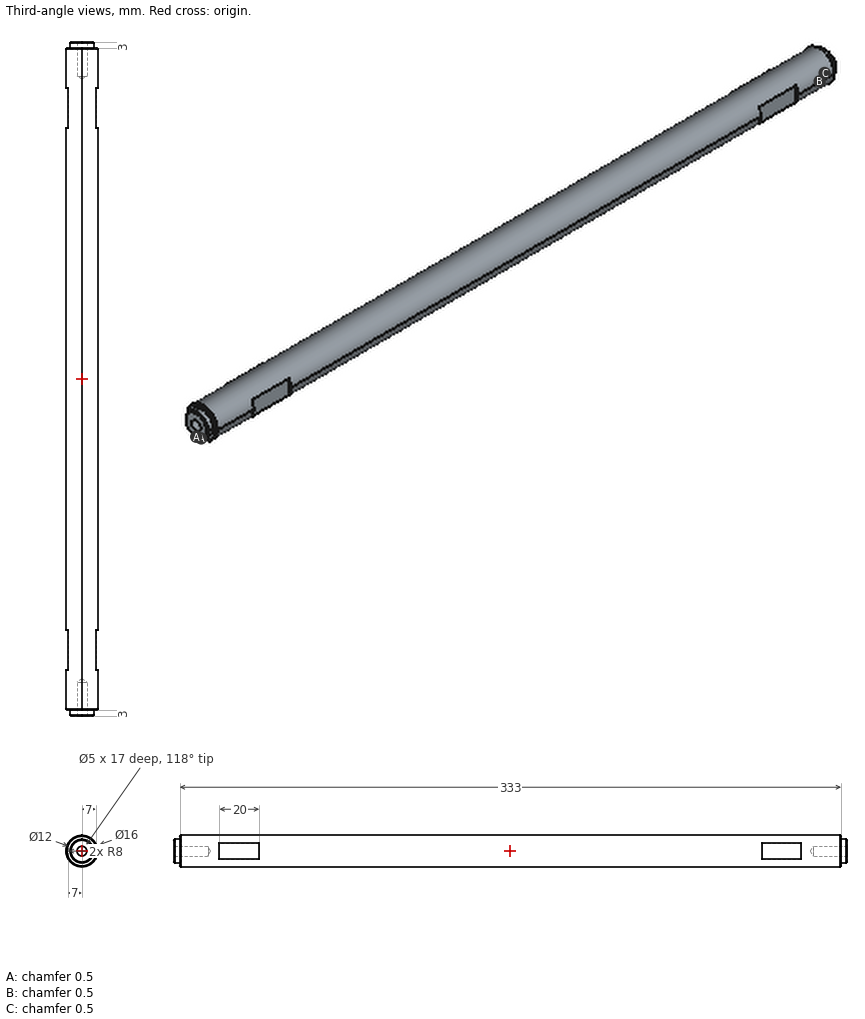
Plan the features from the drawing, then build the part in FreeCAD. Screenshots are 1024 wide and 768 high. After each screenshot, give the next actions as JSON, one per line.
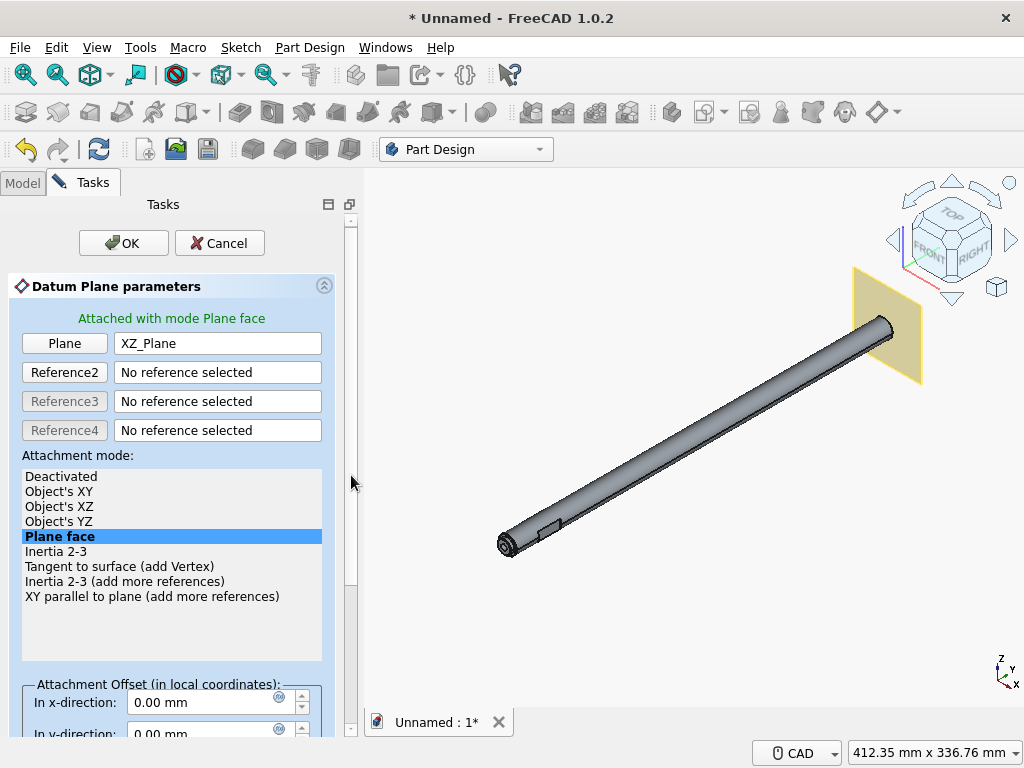
{"action": "left_click", "coordinate": [124, 243]}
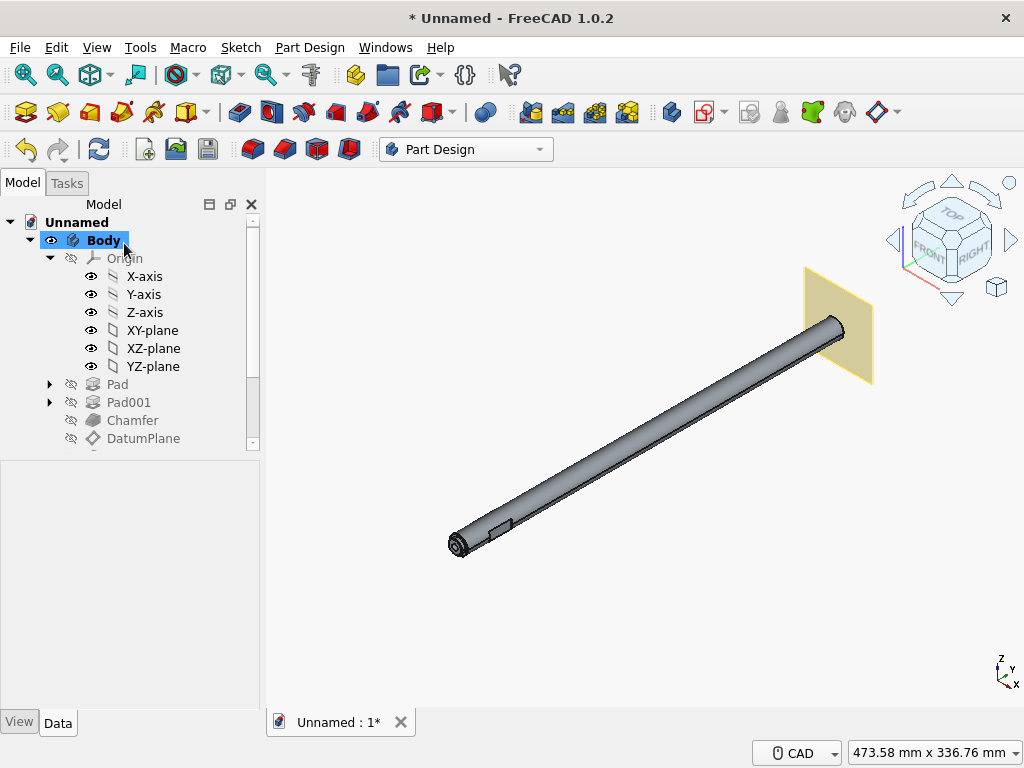
{"action": "scroll", "coordinate": [100, 326], "scroll_direction": "down", "scroll_amount": 3}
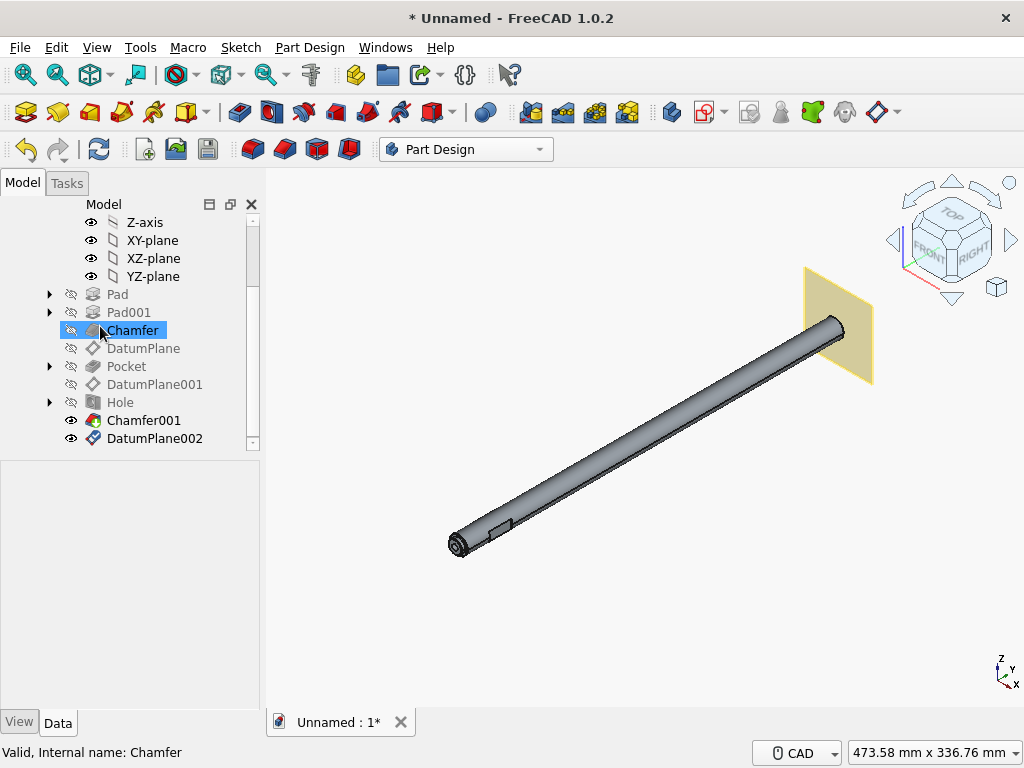
{"action": "left_click", "coordinate": [116, 438]}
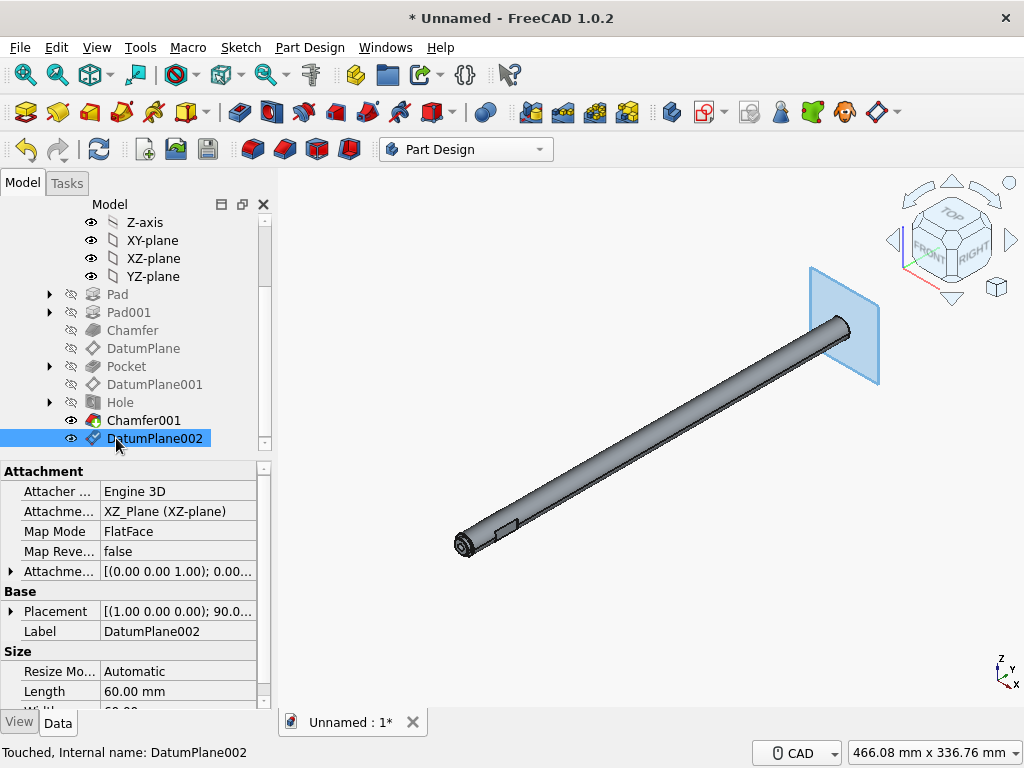
{"action": "left_click", "coordinate": [704, 112]}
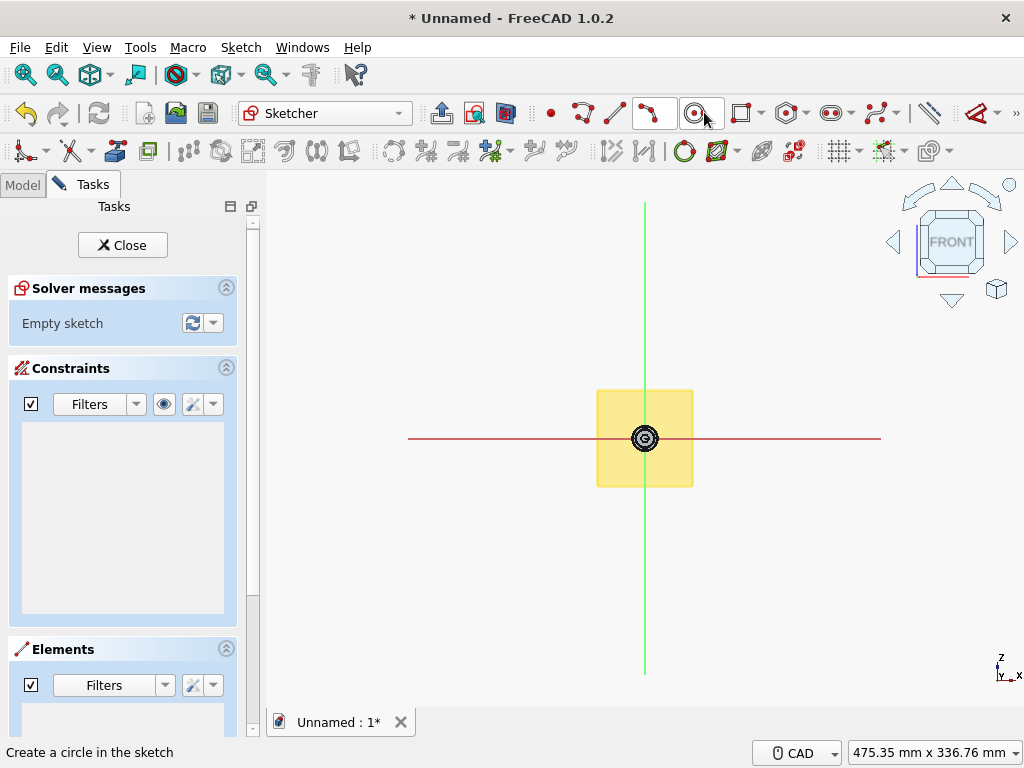
{"action": "key", "text": "q s"}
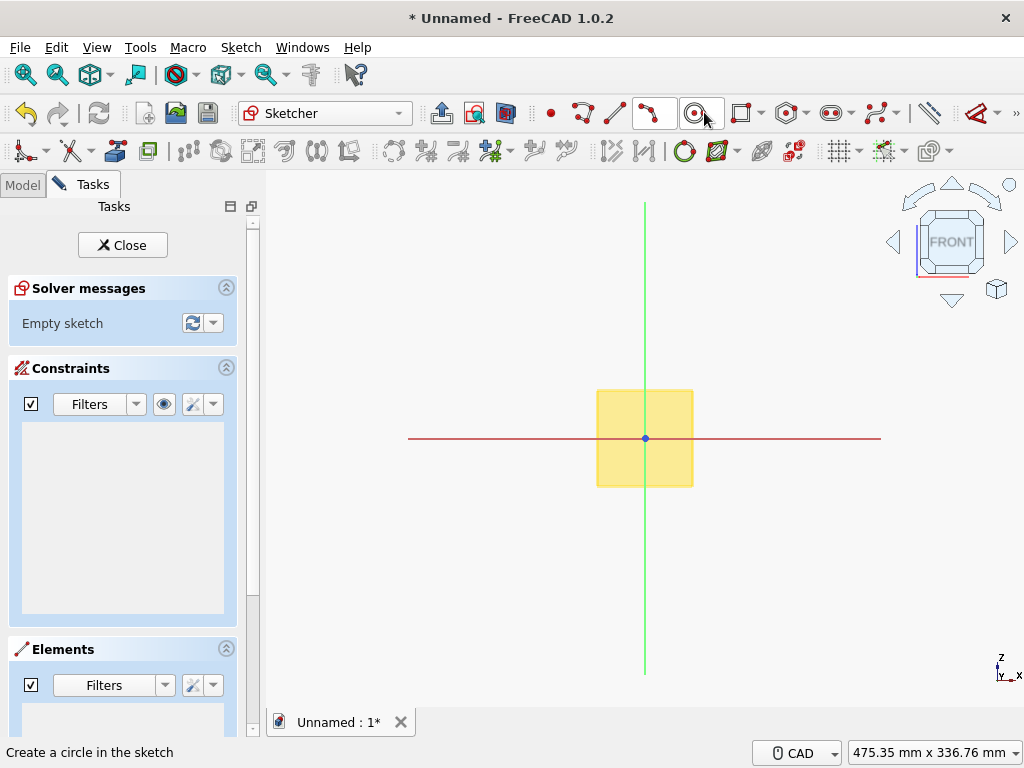
{"action": "scroll", "coordinate": [649, 439], "scroll_direction": "up", "scroll_amount": 14}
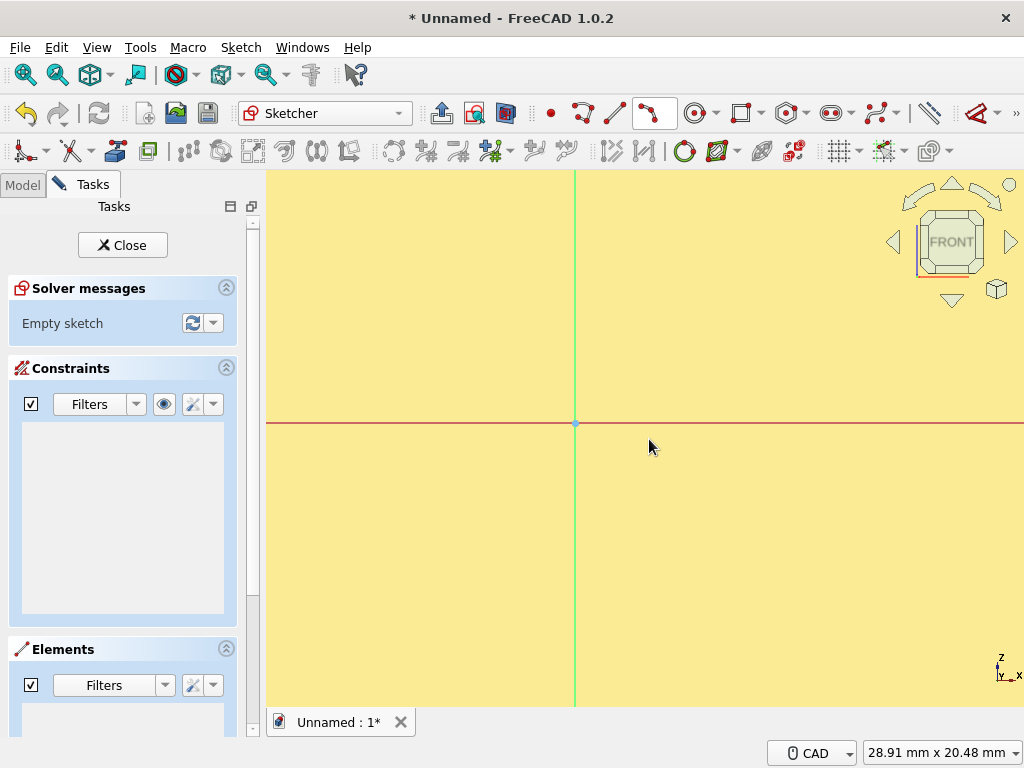
{"action": "left_click", "coordinate": [696, 114]}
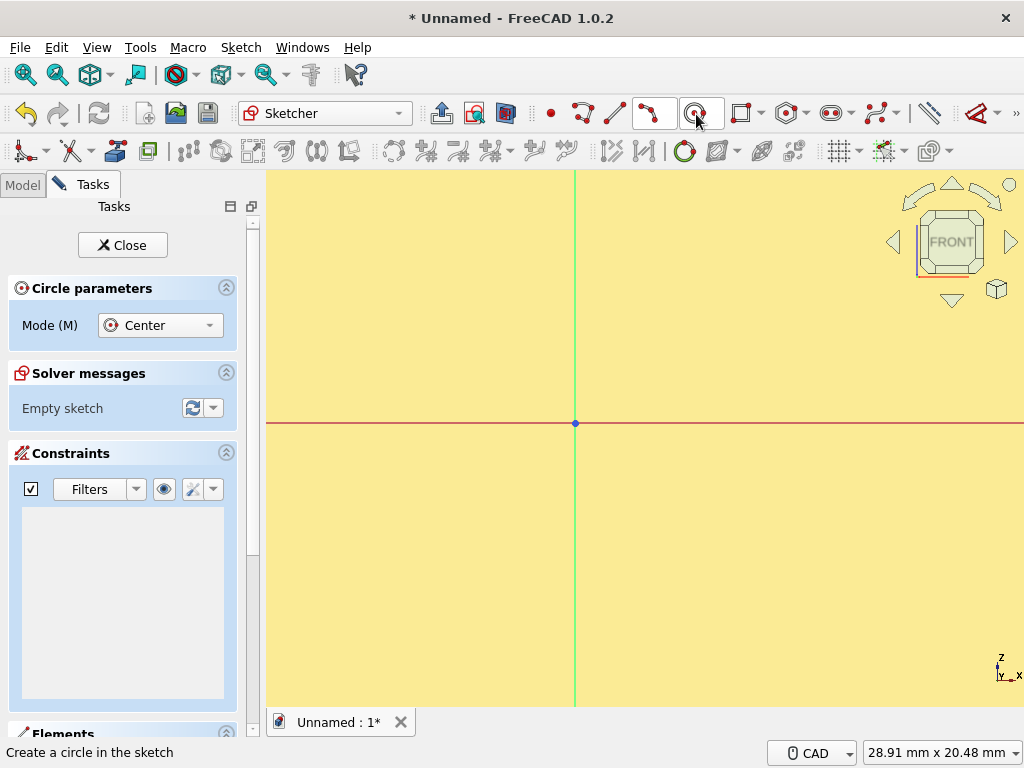
{"action": "left_click", "coordinate": [575, 423]}
{"action": "left_click", "coordinate": [687, 312]}
{"action": "key", "text": "Escape"}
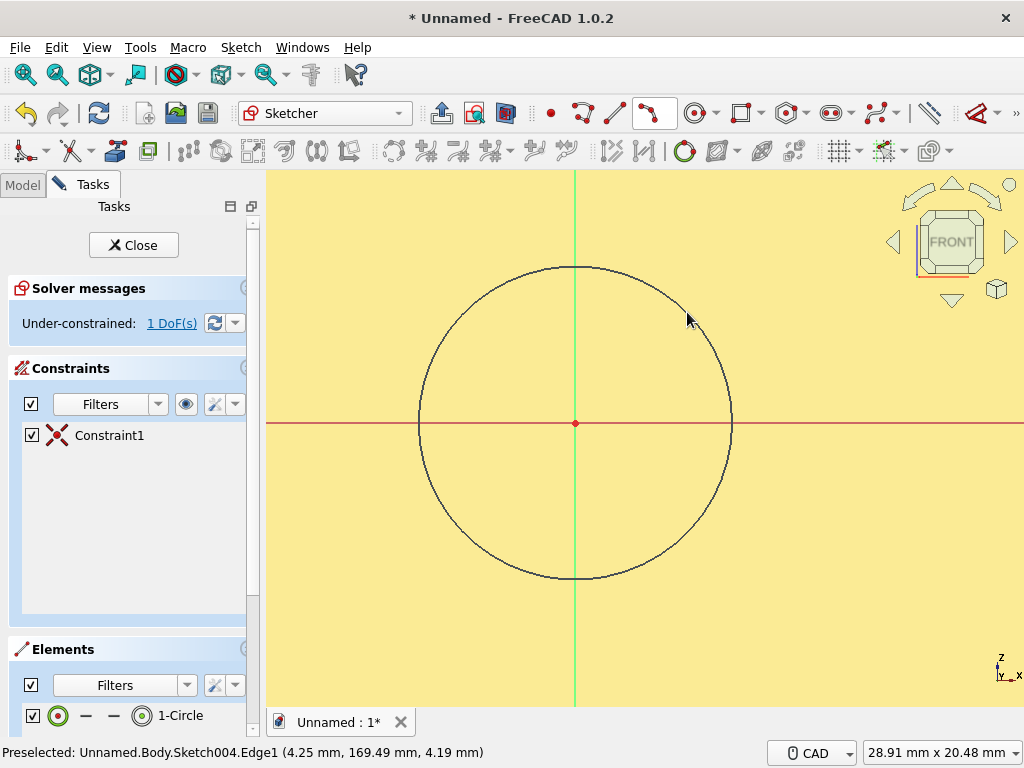
{"action": "left_click", "coordinate": [976, 114]}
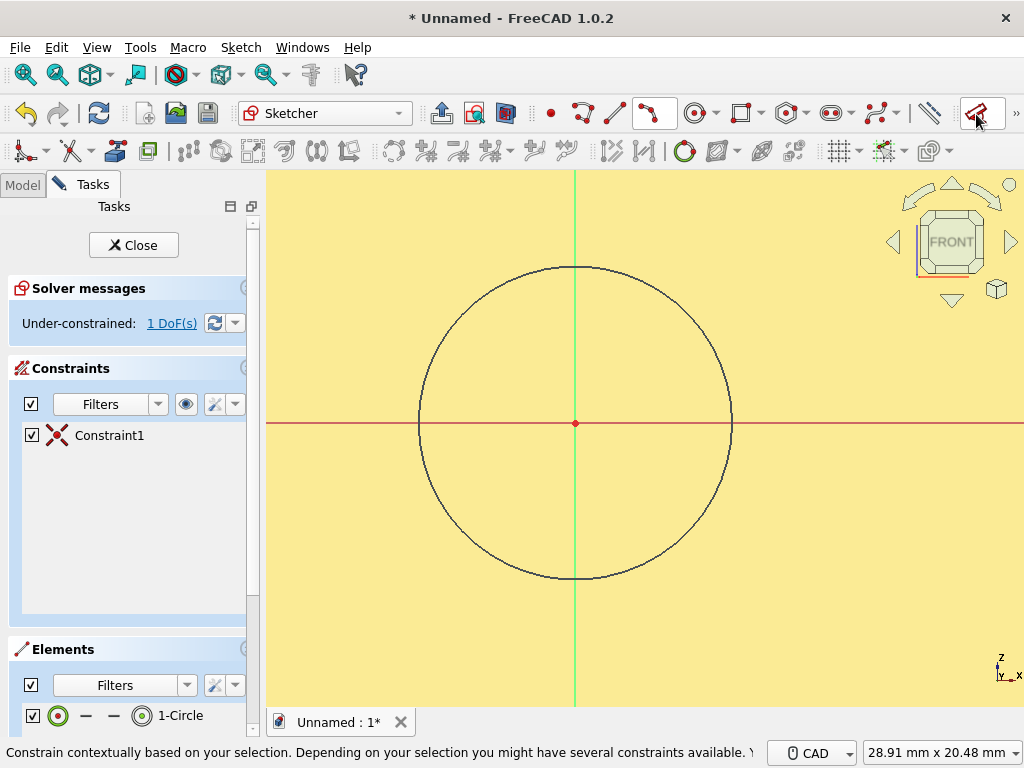
{"action": "left_click", "coordinate": [686, 312]}
{"action": "left_click", "coordinate": [709, 289]}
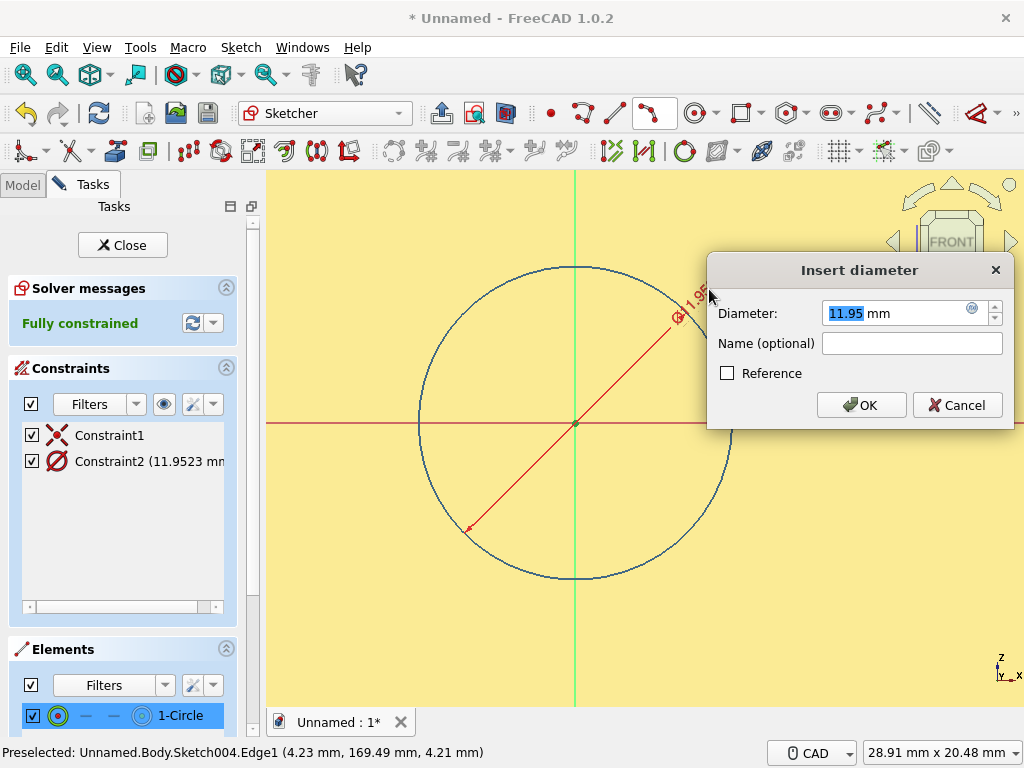
{"action": "type", "text": "12"}
{"action": "key", "text": "Return"}
{"action": "key", "text": "Escape"}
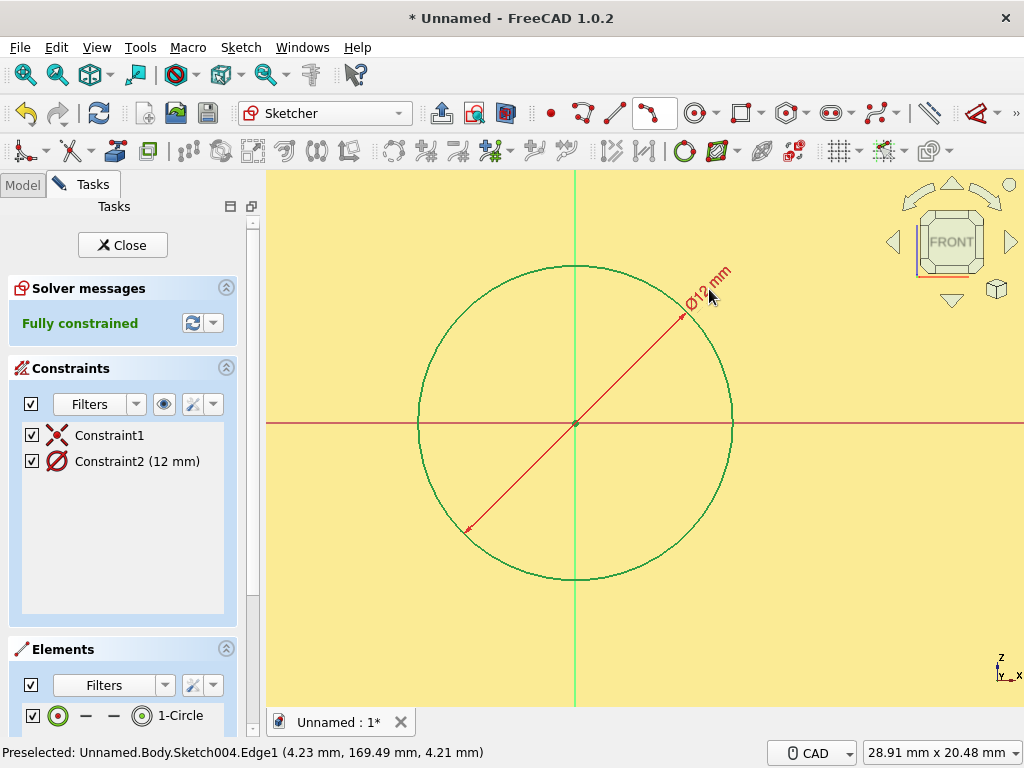
{"action": "left_click", "coordinate": [123, 245]}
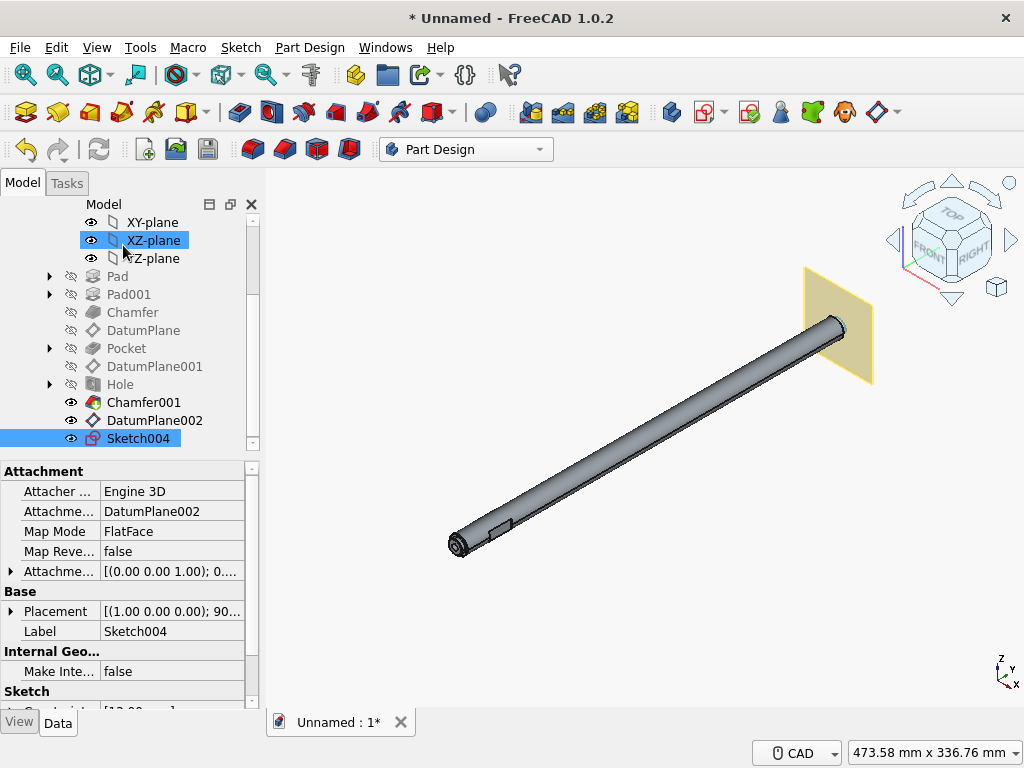
{"action": "left_click", "coordinate": [26, 112]}